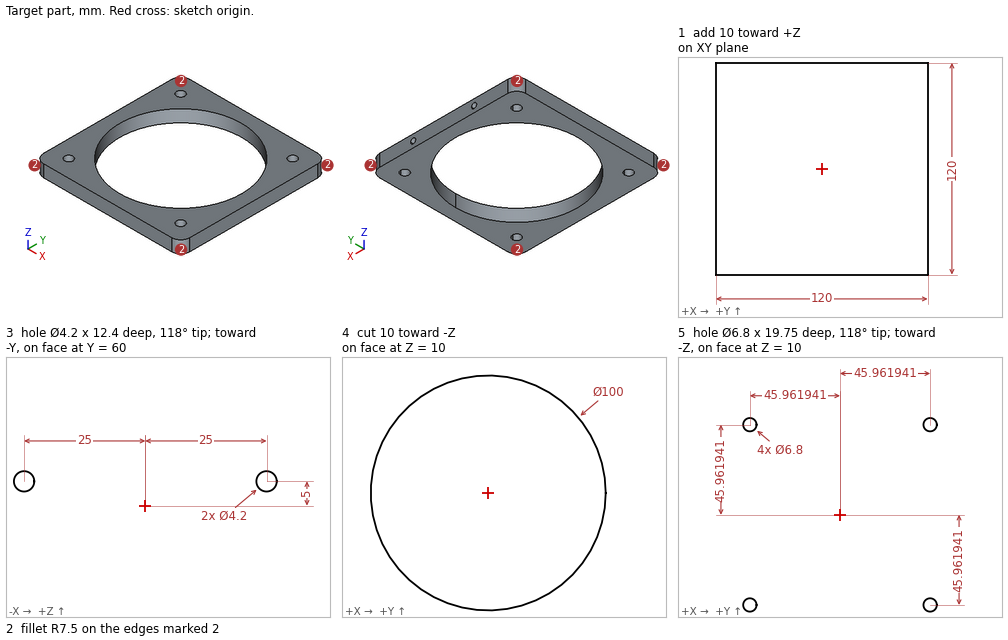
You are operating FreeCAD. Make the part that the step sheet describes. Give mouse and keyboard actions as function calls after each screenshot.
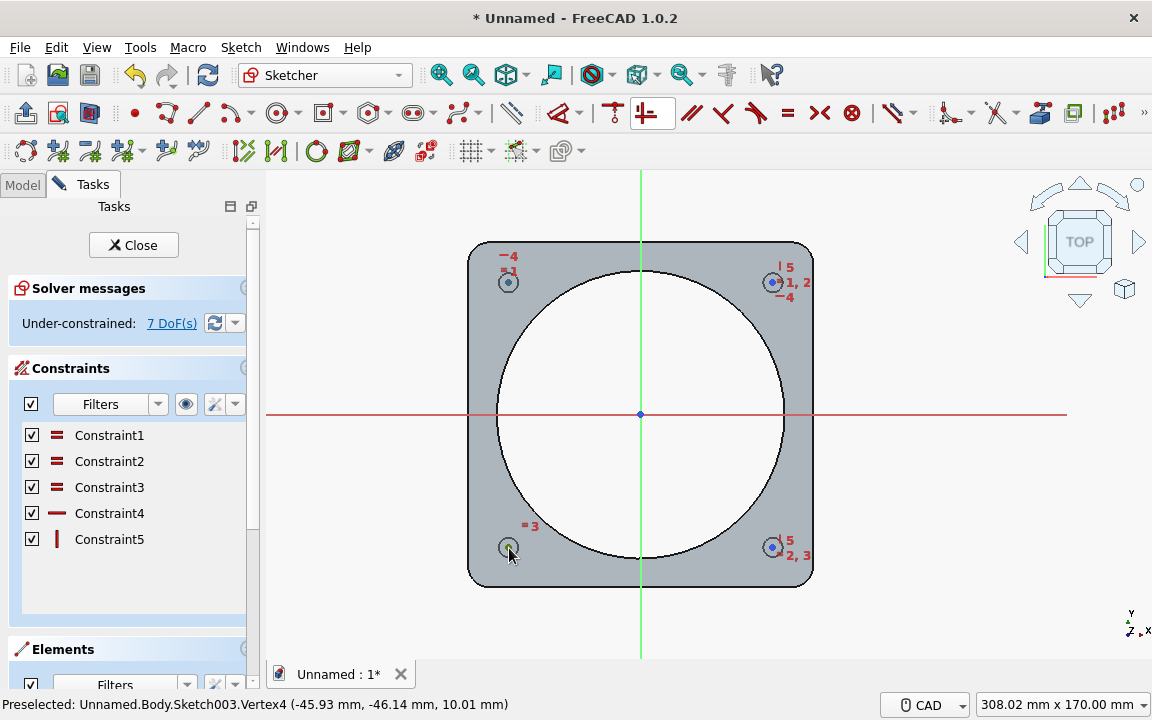
key(v)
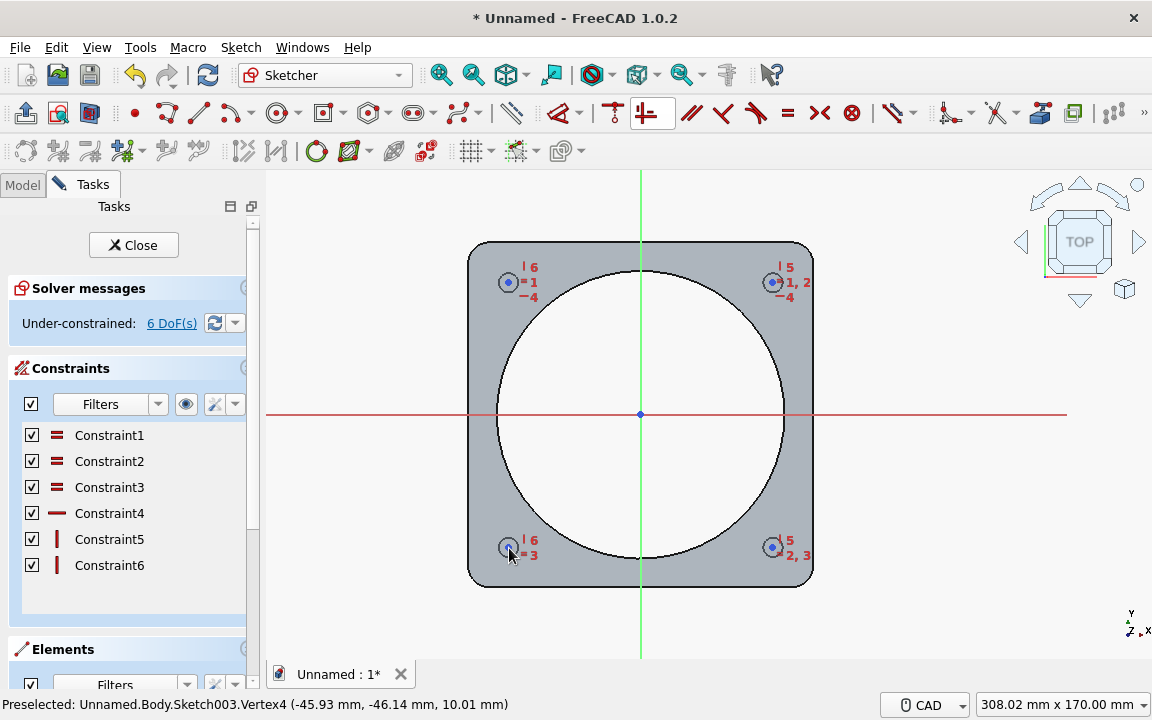
click(773, 547)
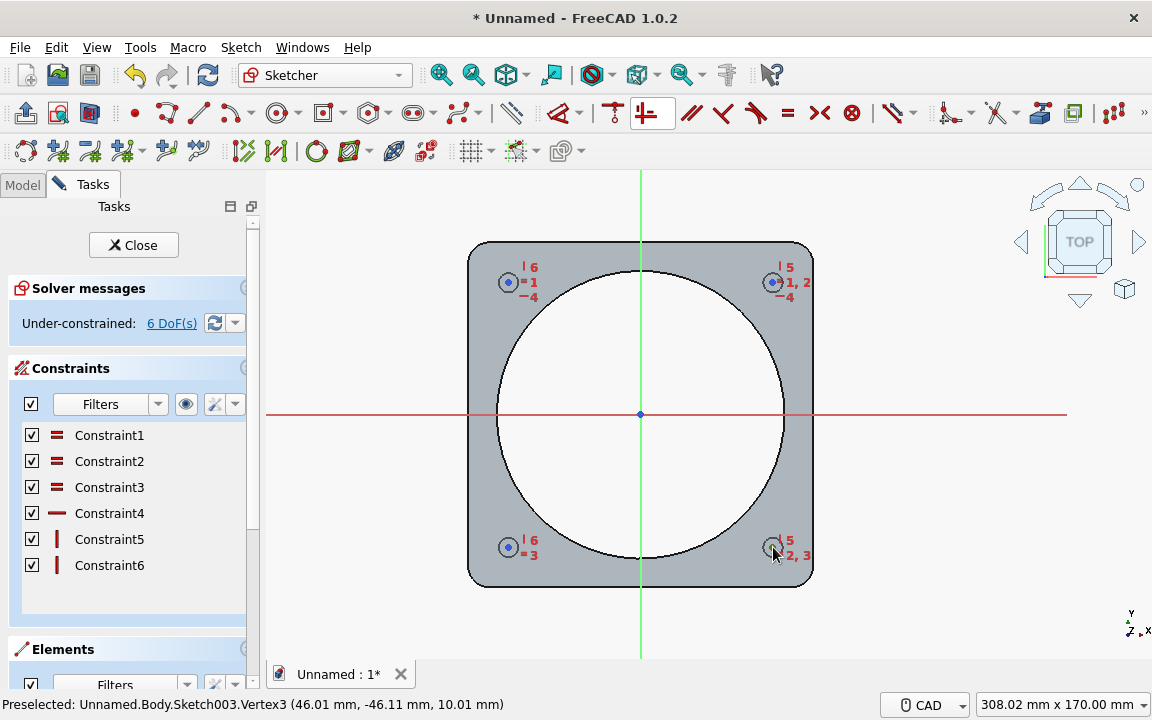
click(509, 548)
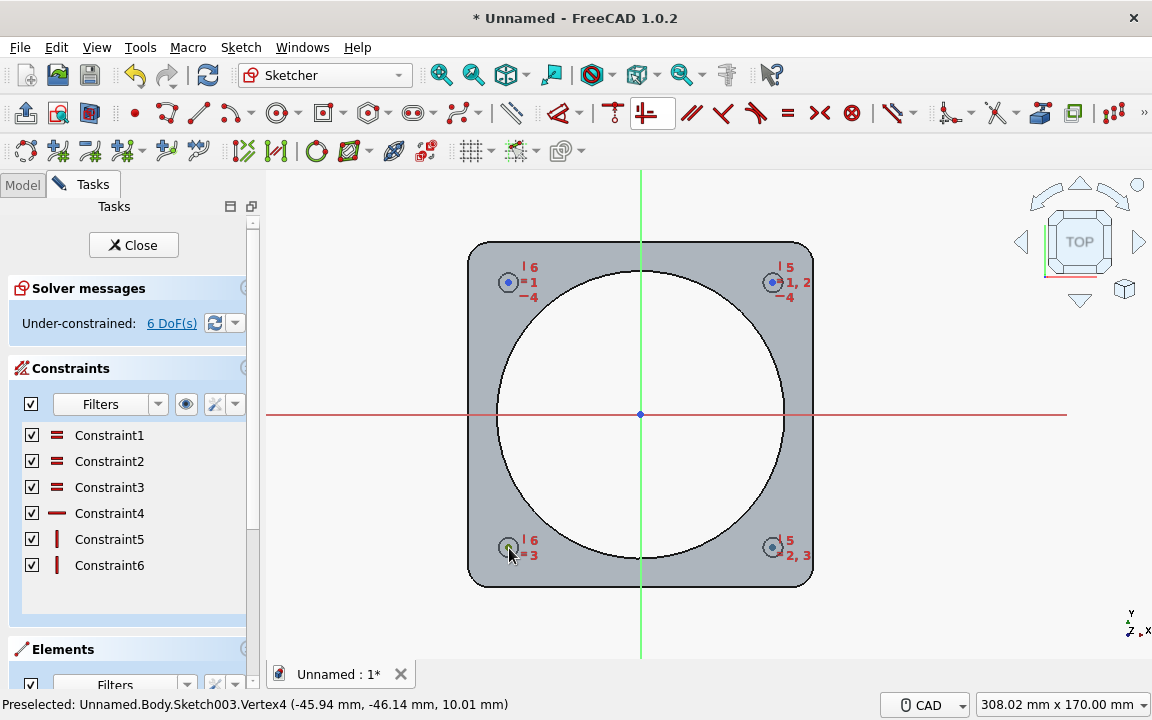
click(670, 114)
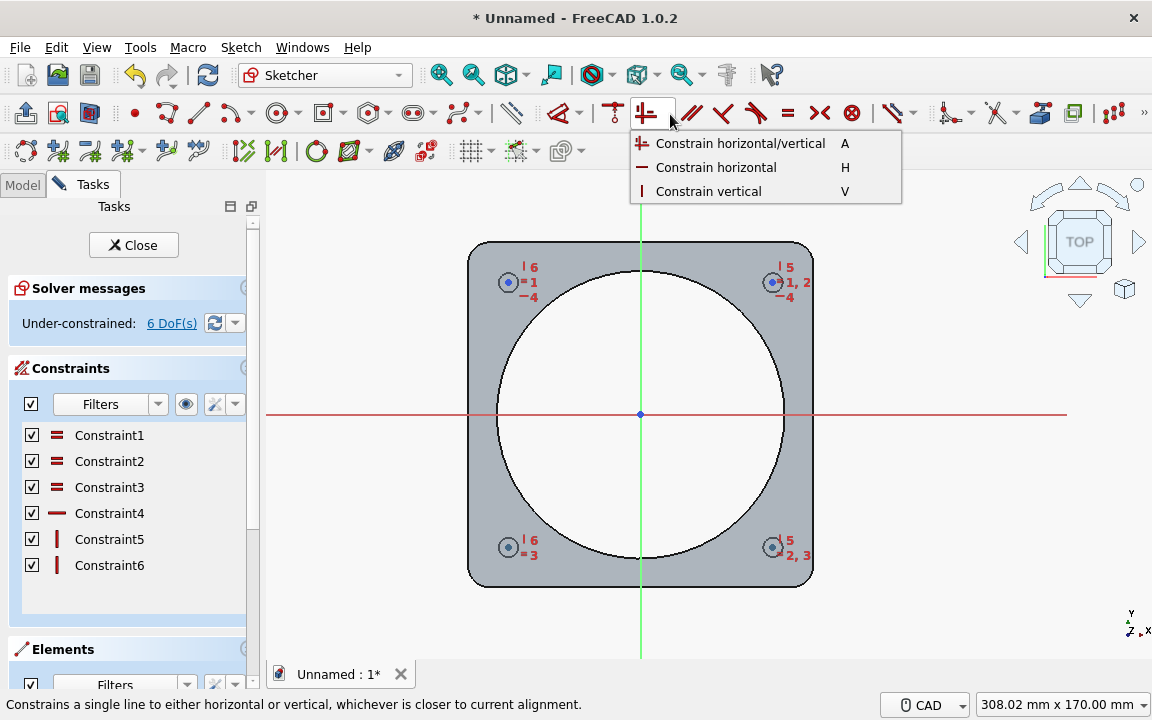
click(766, 167)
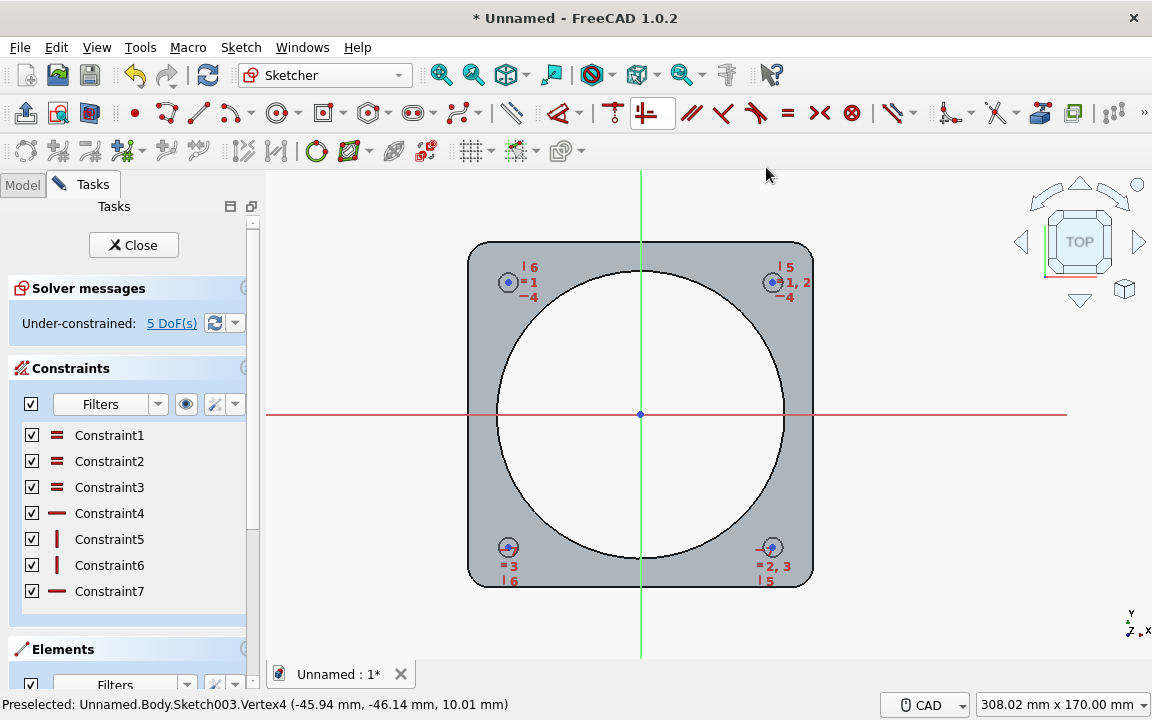
click(558, 114)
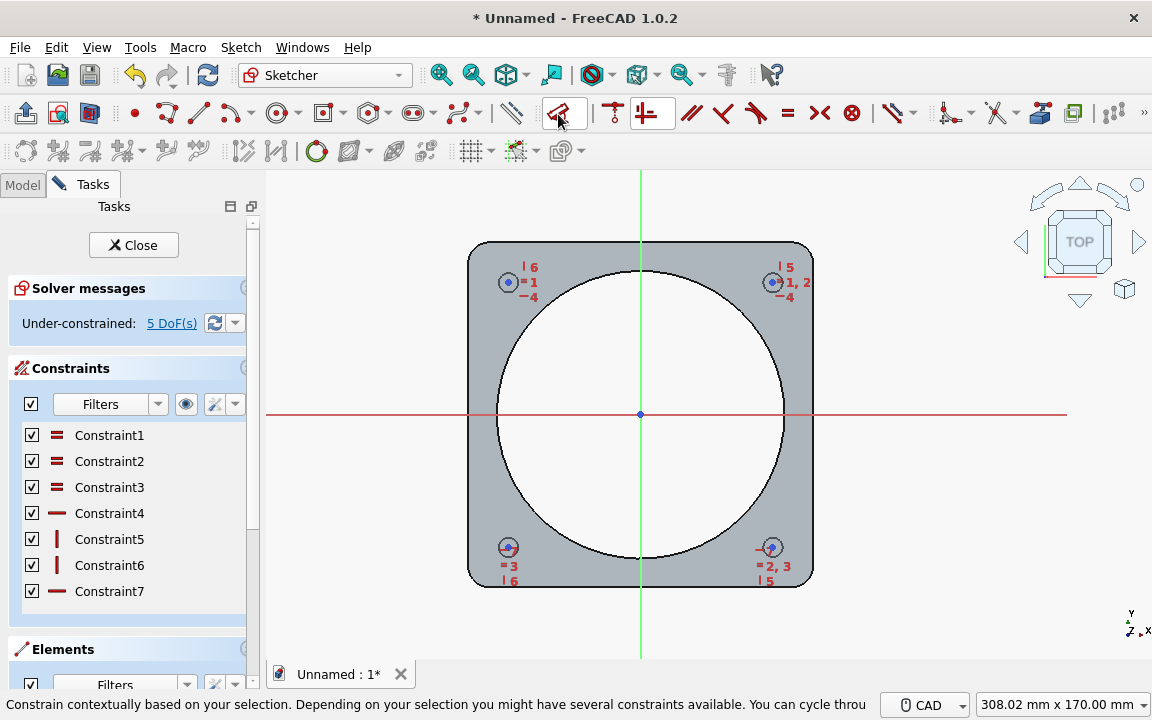
scroll(515, 276, up, 4)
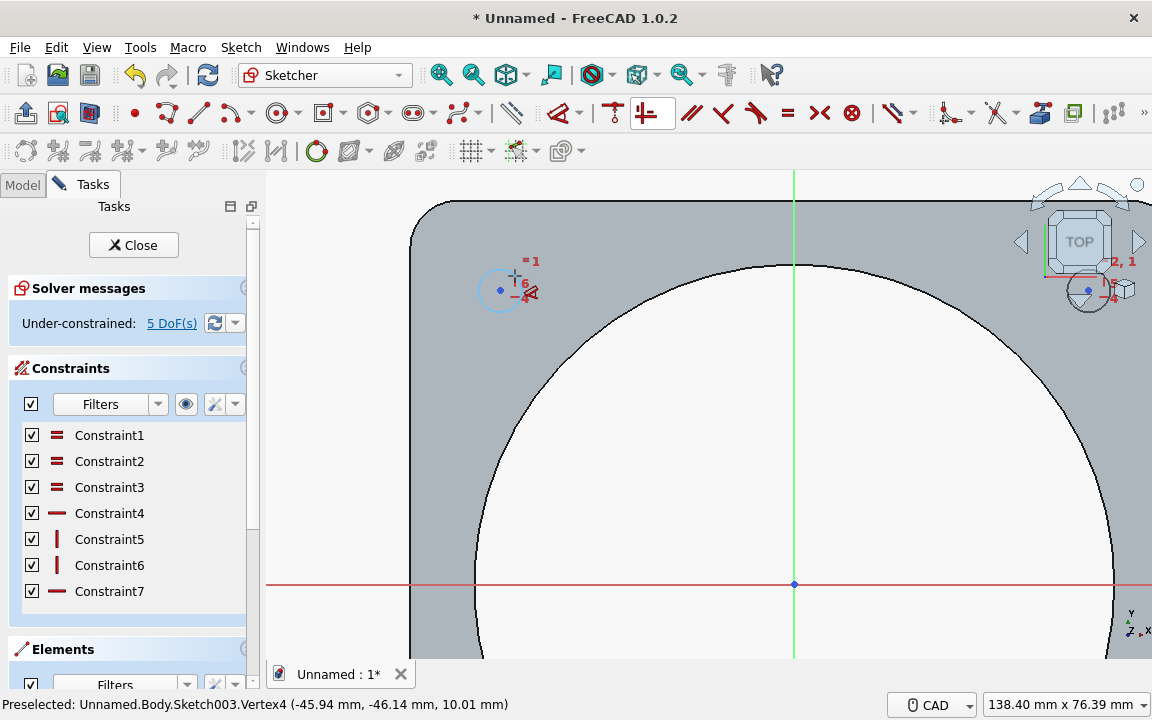
click(515, 276)
click(538, 253)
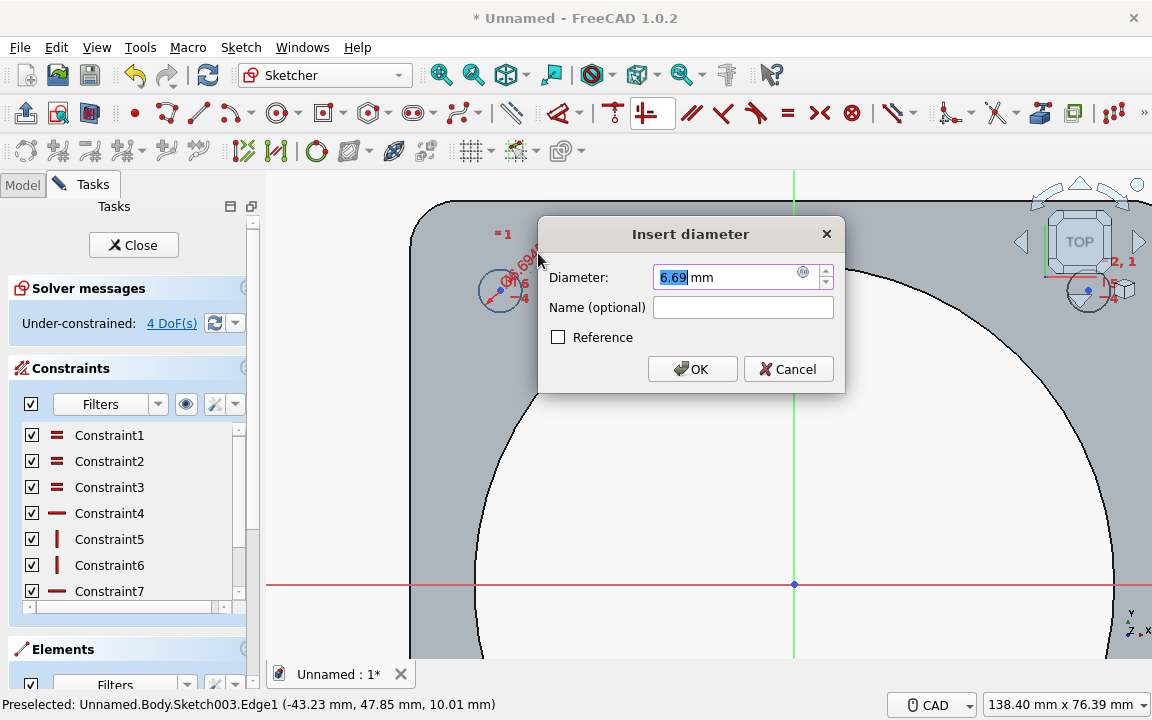
text(6.8)
key(Return)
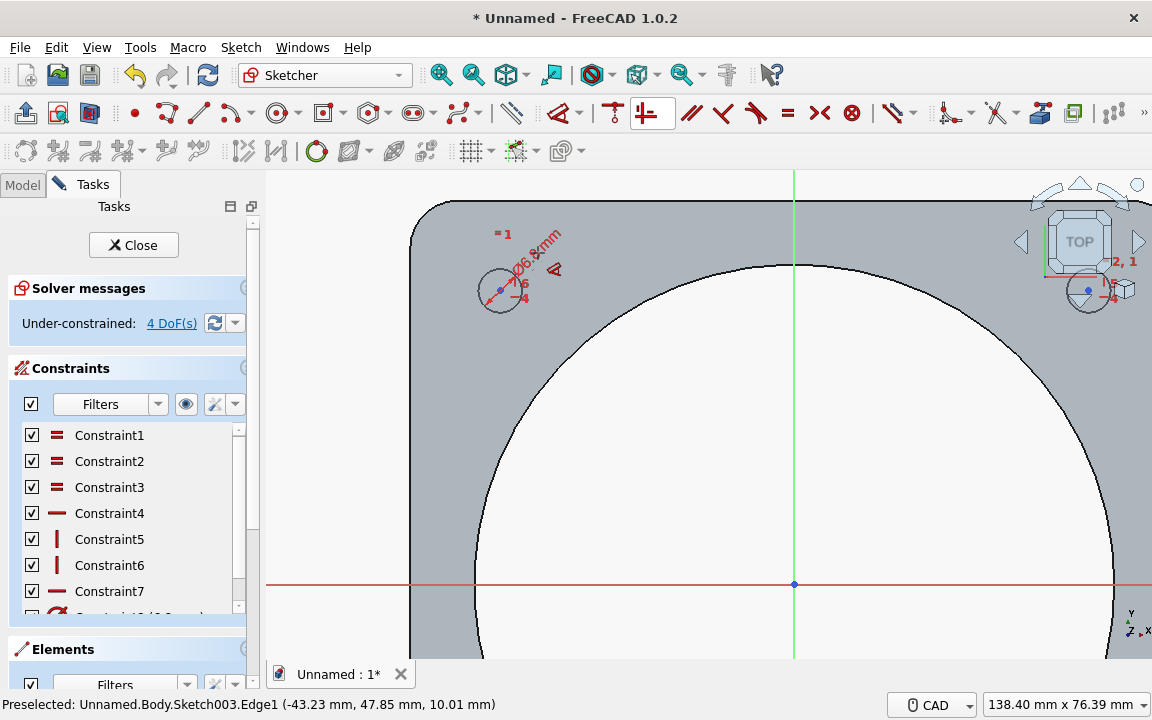
click(500, 291)
click(647, 257)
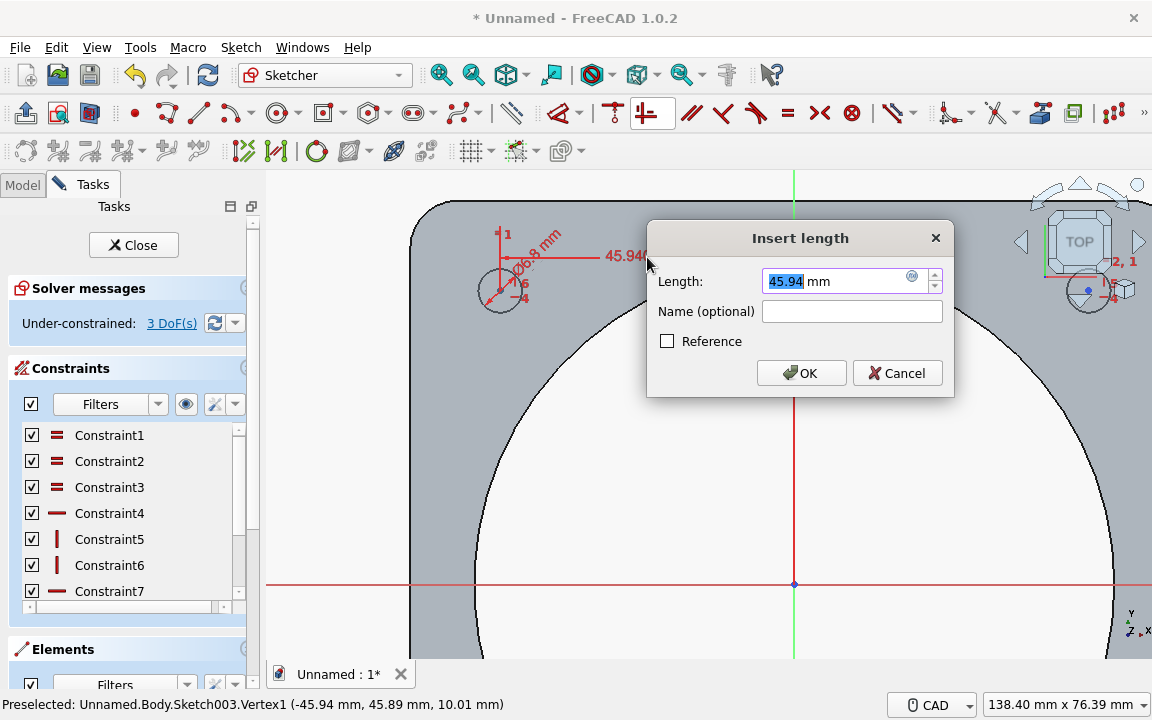
text(45.961941)
key(Return)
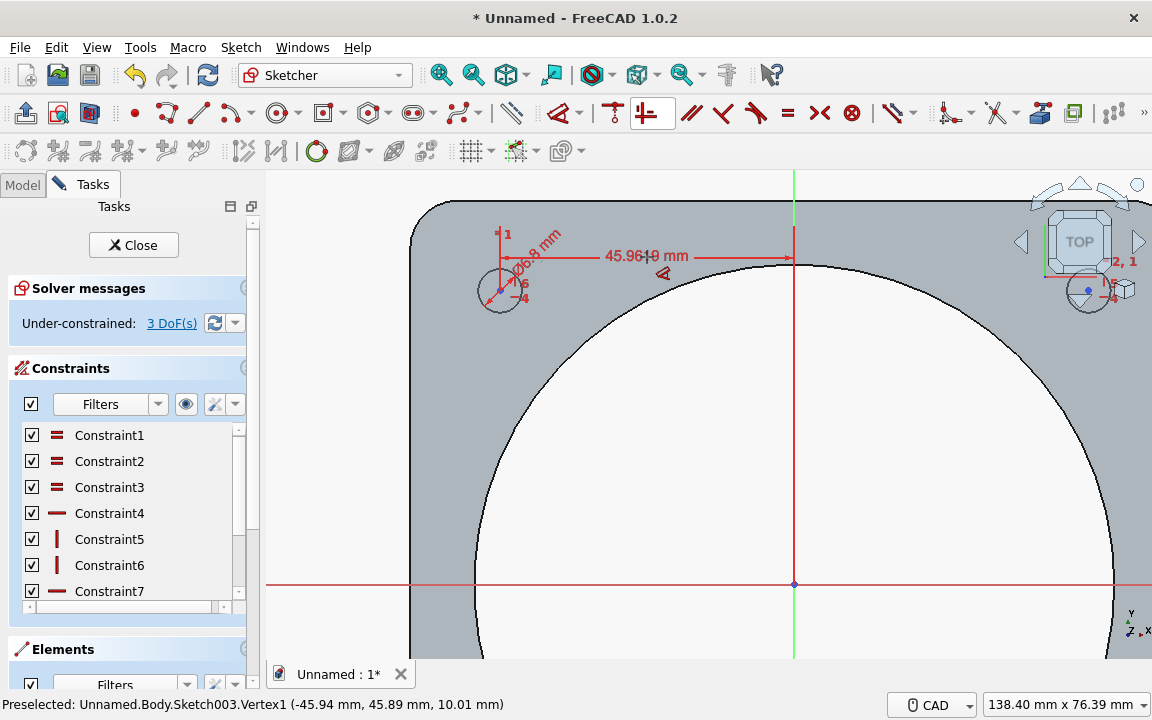
click(500, 291)
click(466, 438)